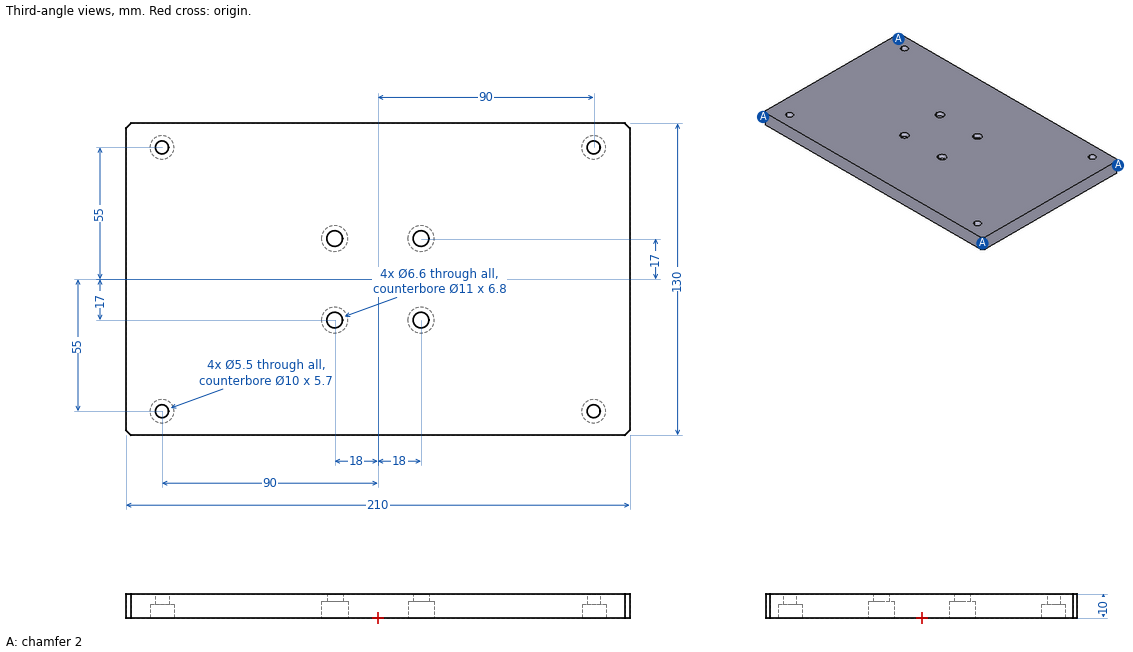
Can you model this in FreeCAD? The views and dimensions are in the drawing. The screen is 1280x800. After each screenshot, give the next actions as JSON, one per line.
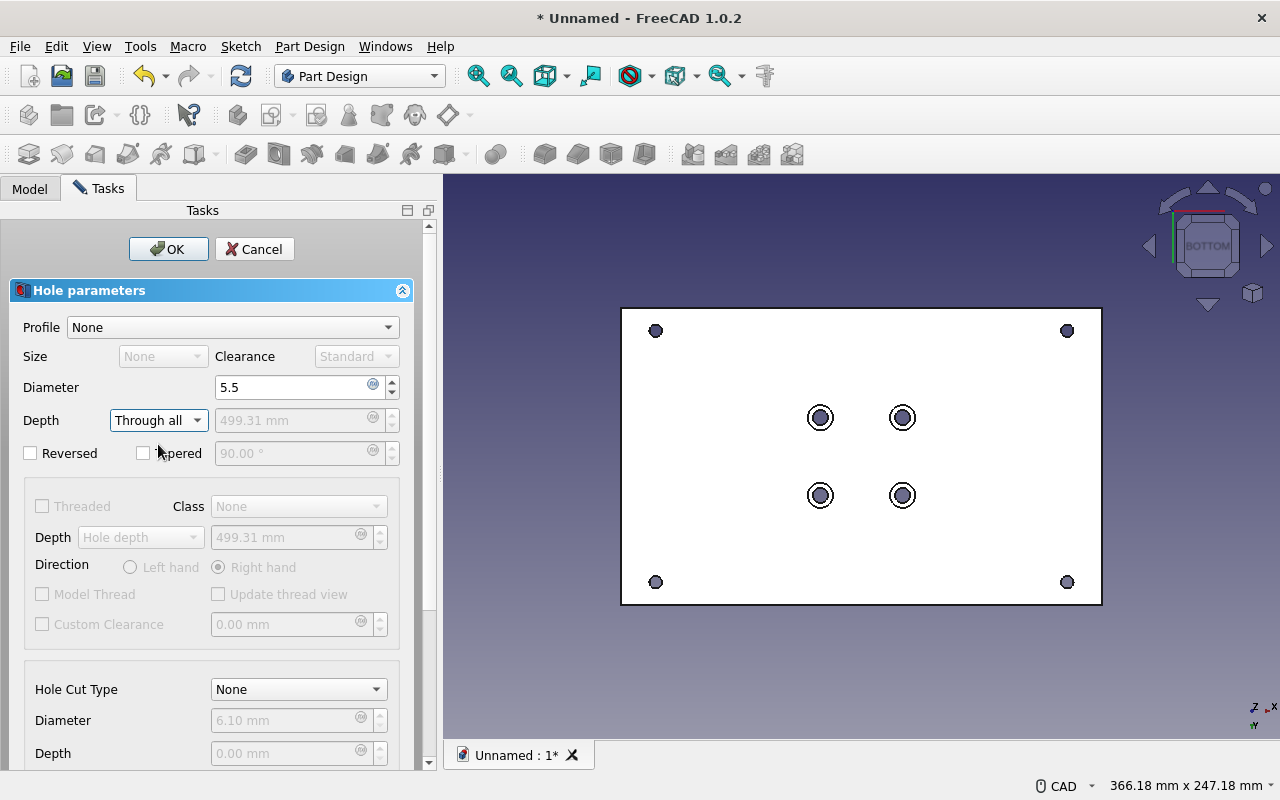
{"action": "left_click", "coordinate": [300, 690]}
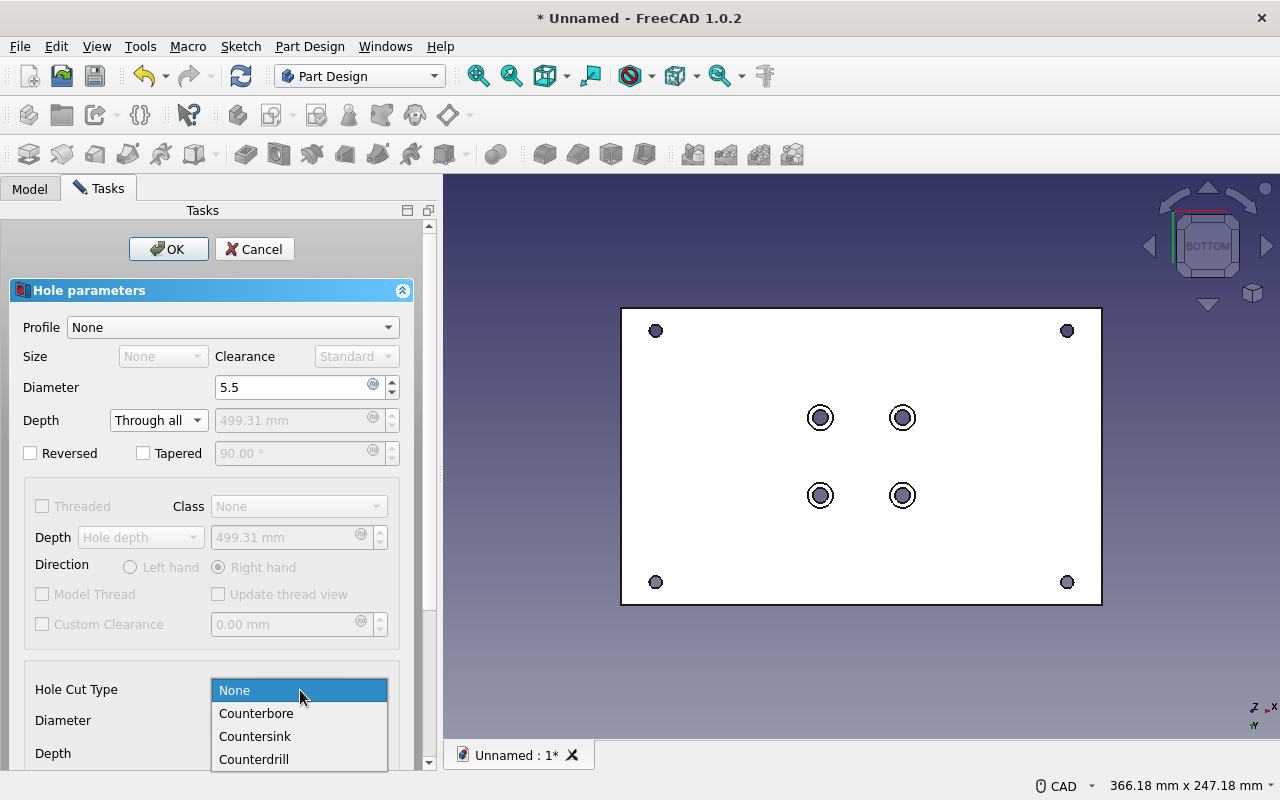
{"action": "left_click", "coordinate": [298, 714]}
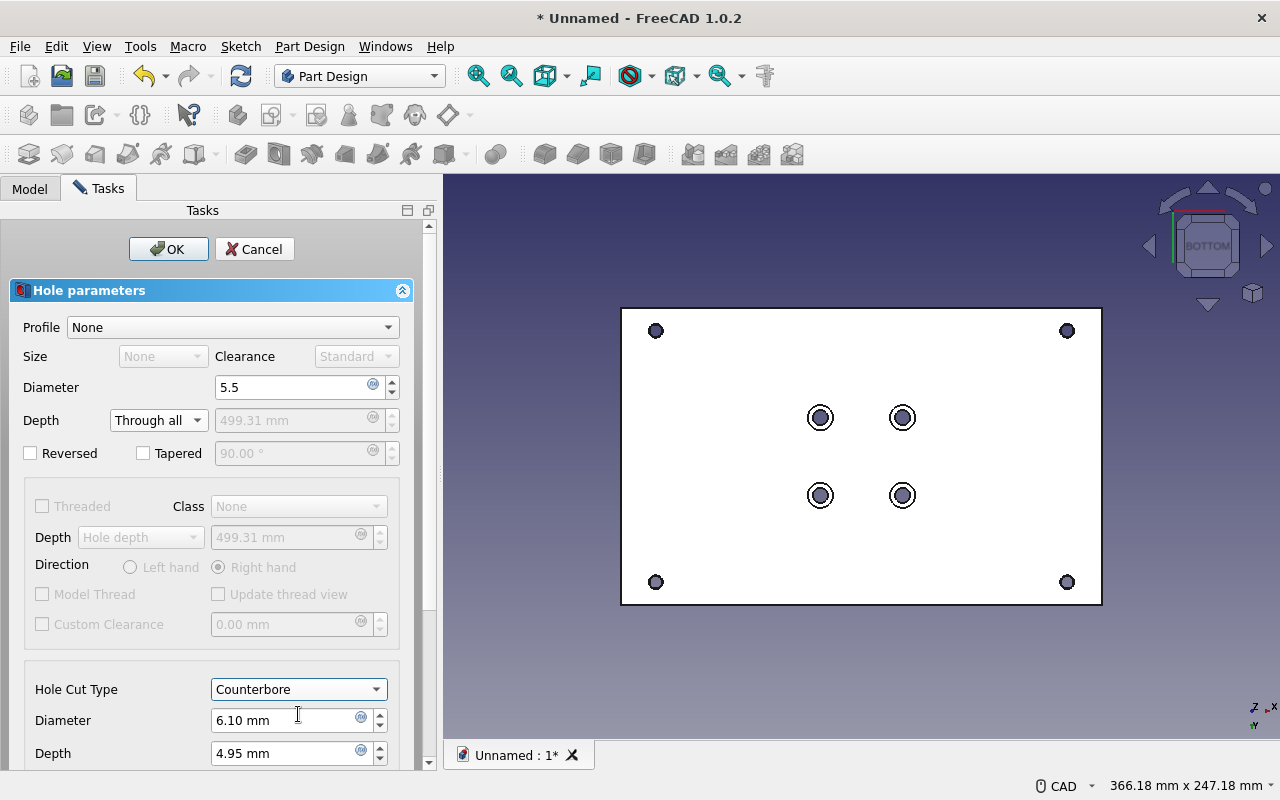
{"action": "triple_click", "coordinate": [292, 720]}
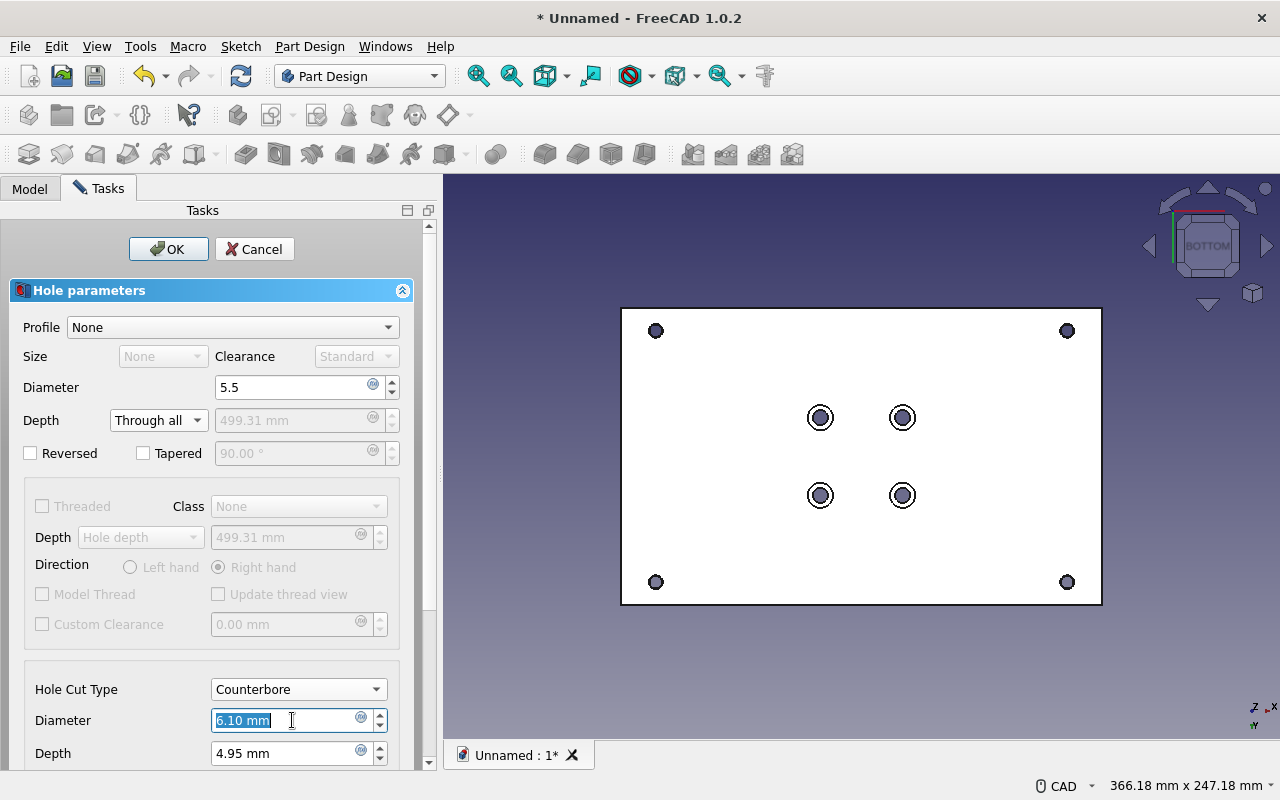
{"action": "type", "text": "10"}
{"action": "key", "text": "Tab"}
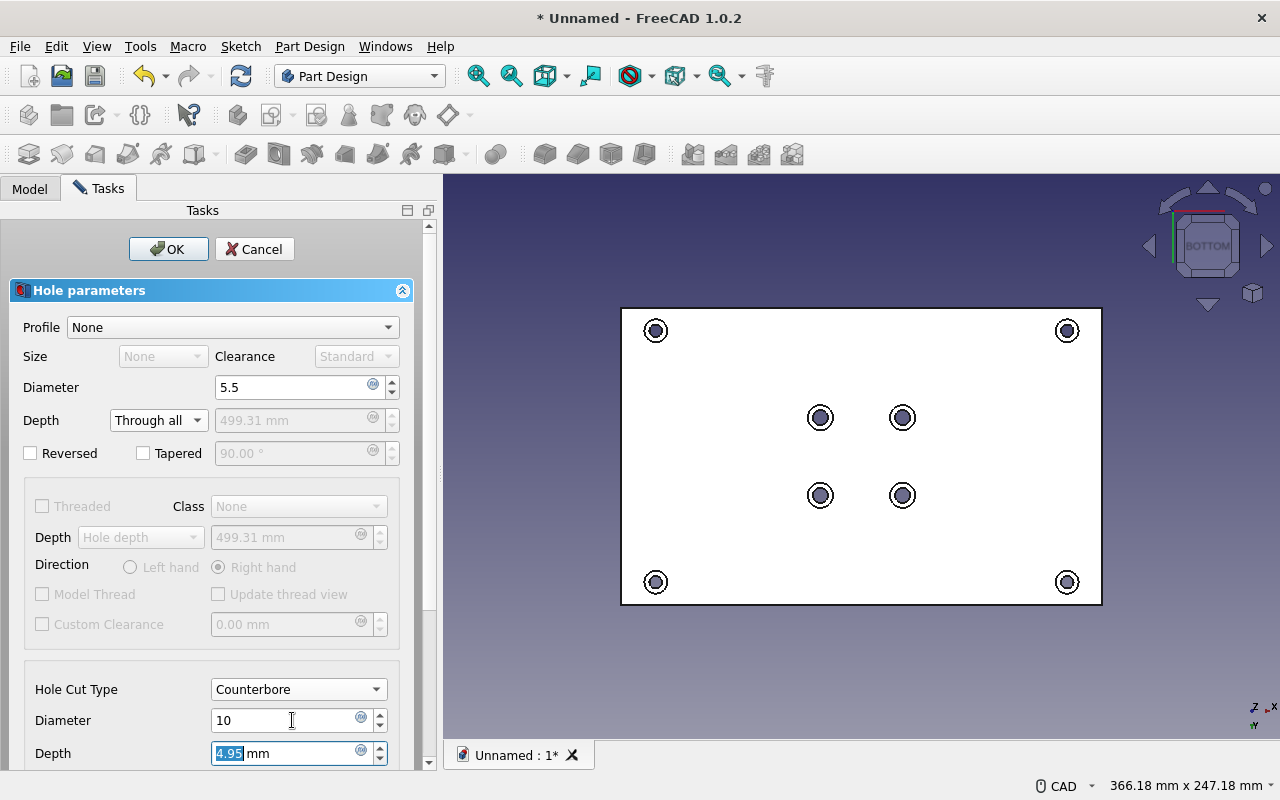
{"action": "type", "text": "5.7"}
{"action": "key", "text": "Tab"}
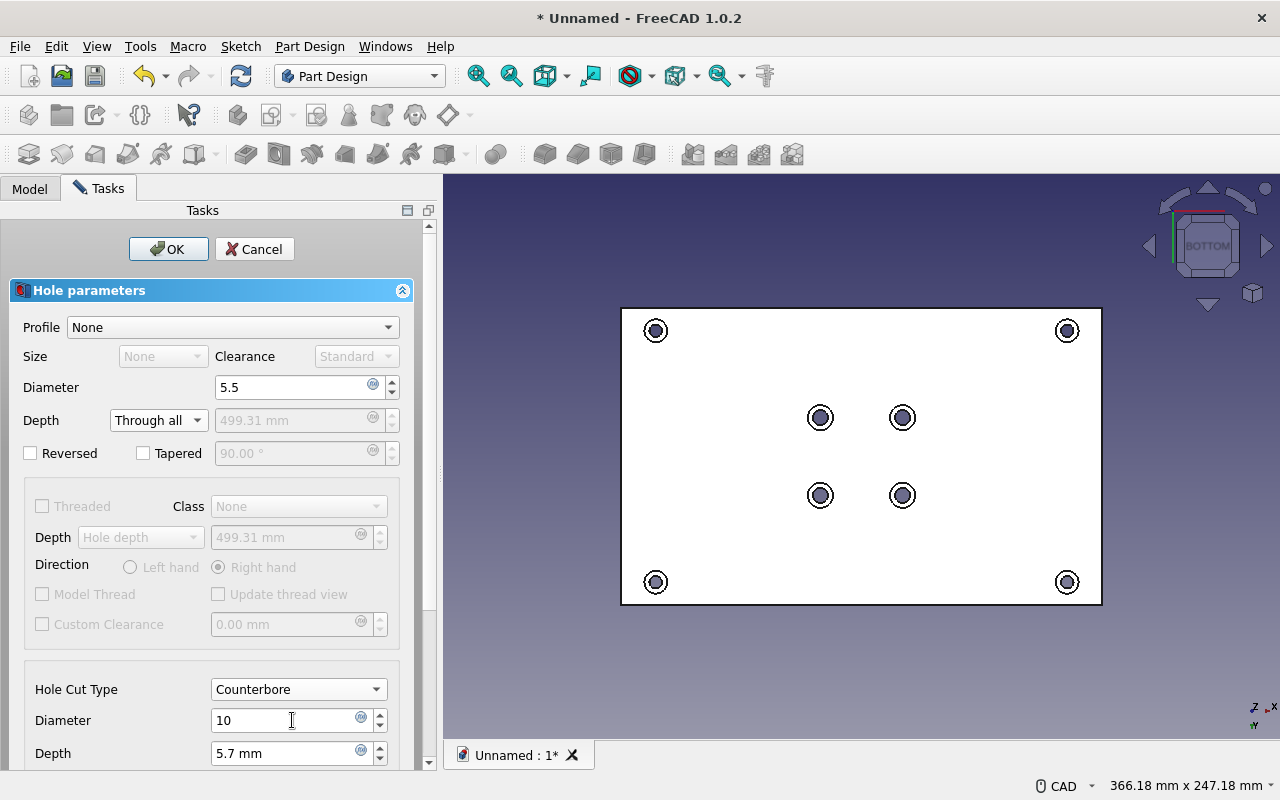
{"action": "left_click", "coordinate": [169, 249]}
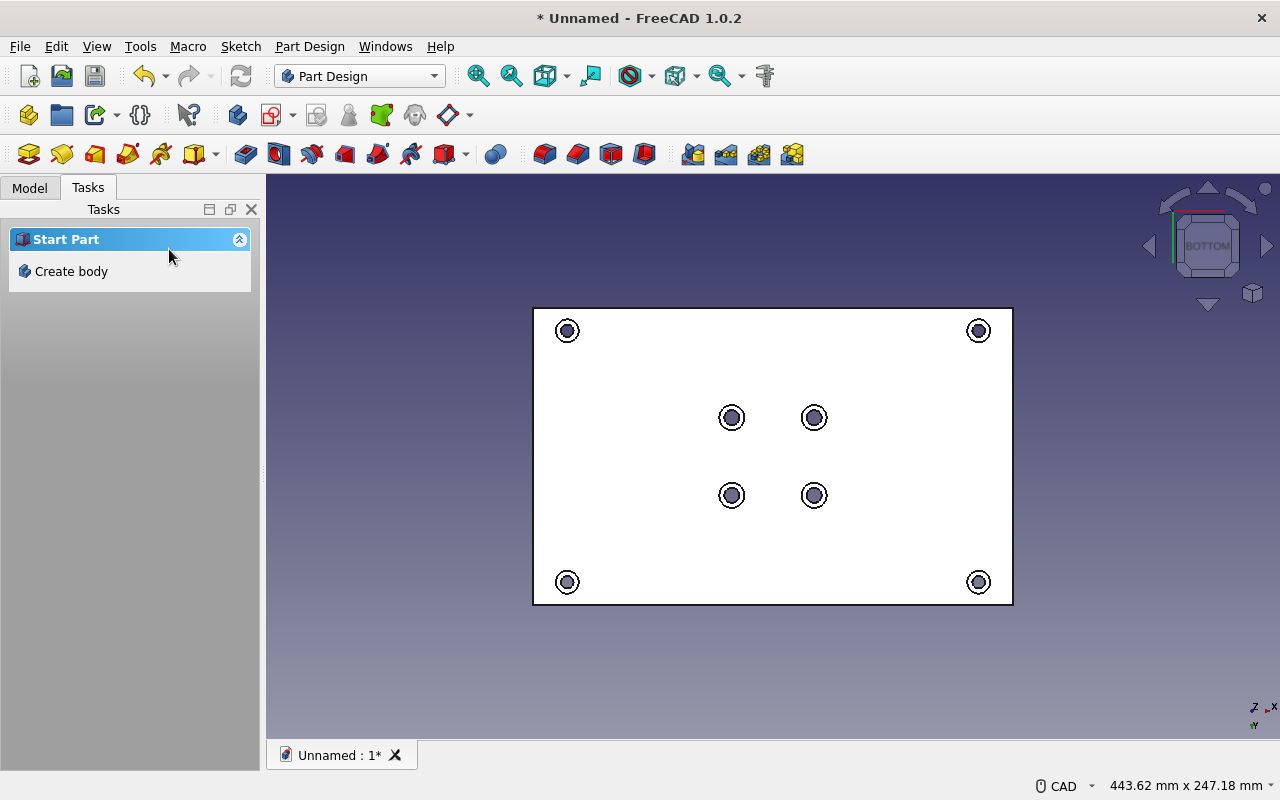
{"action": "key", "text": "0"}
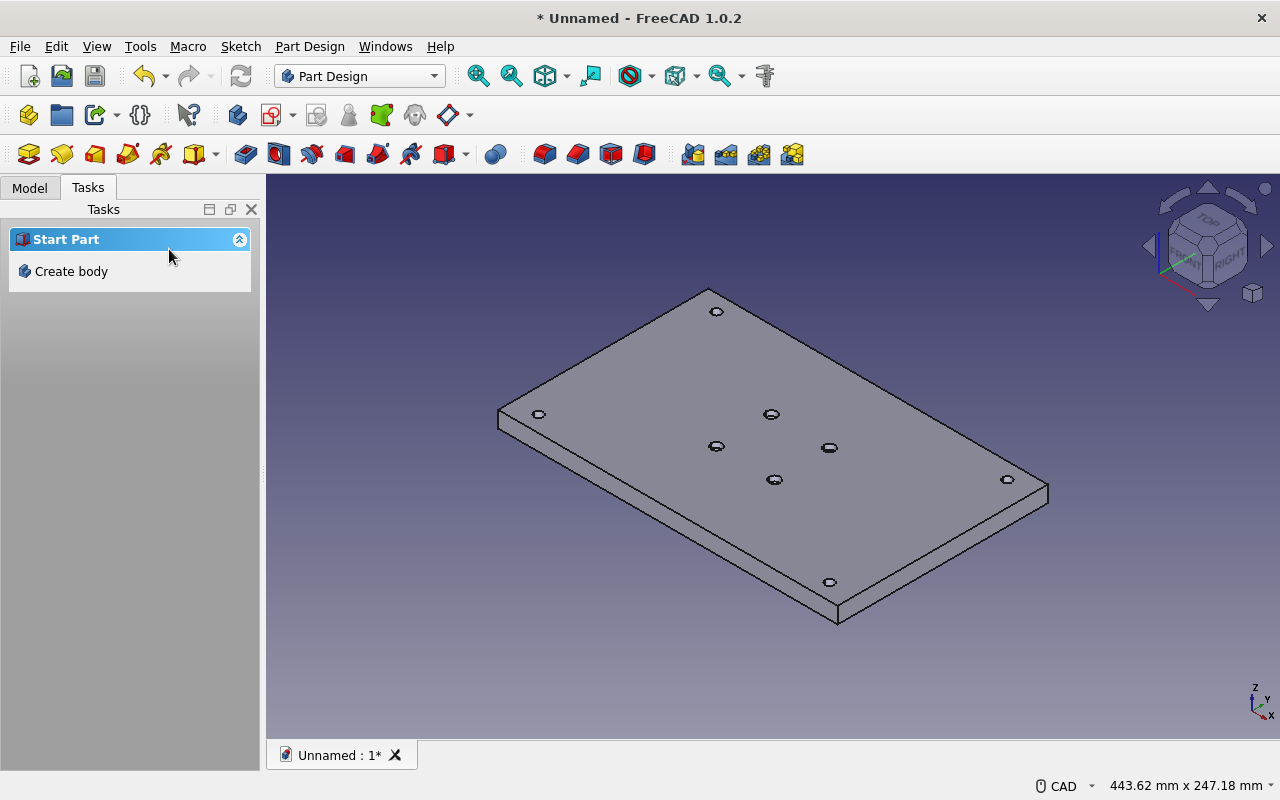
{"action": "left_click", "coordinate": [838, 614]}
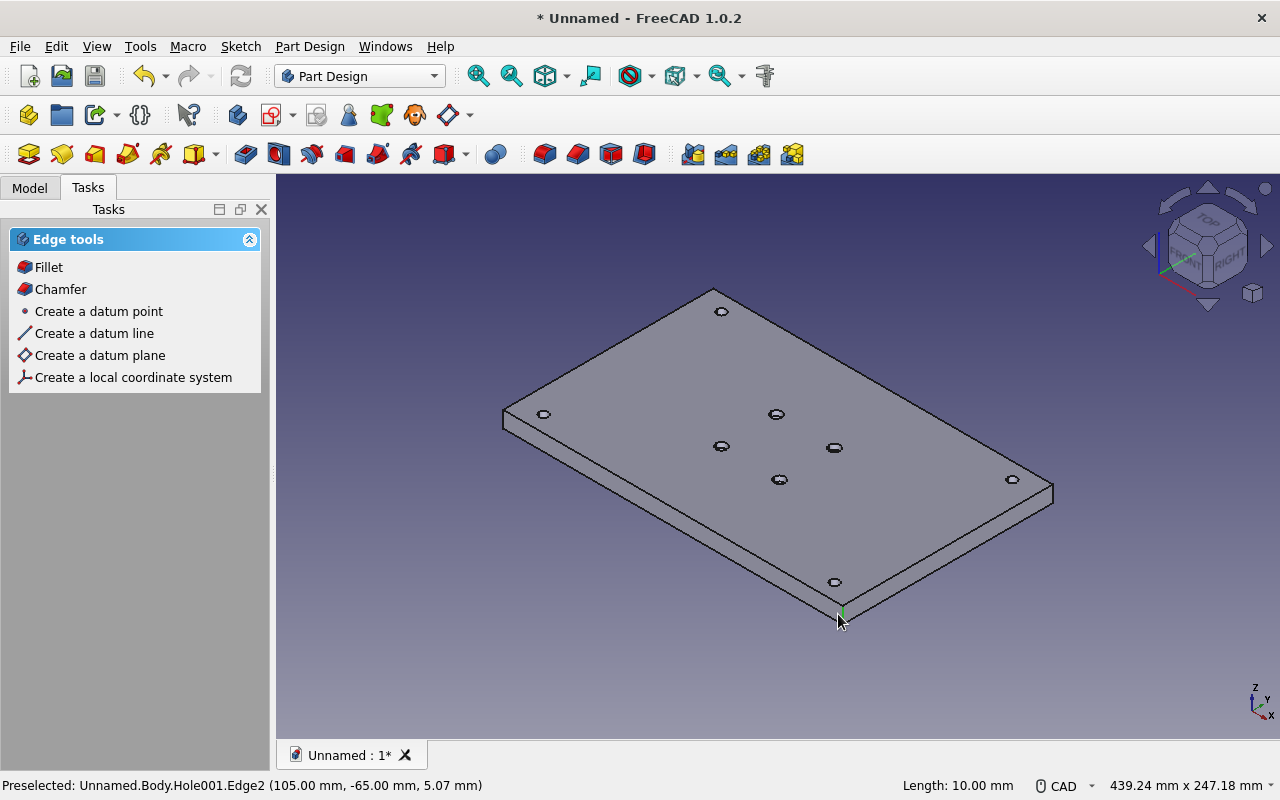
{"action": "key", "text": "2"}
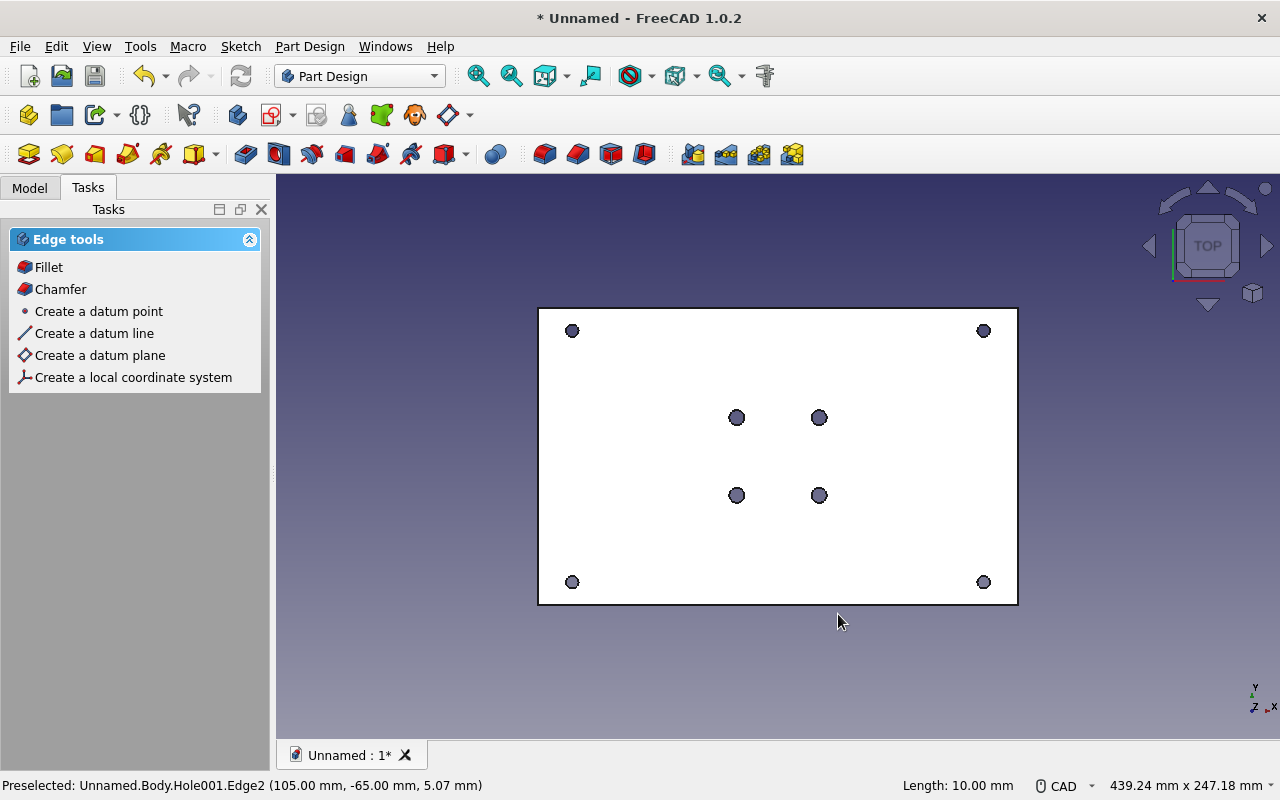
{"action": "key", "text": "1"}